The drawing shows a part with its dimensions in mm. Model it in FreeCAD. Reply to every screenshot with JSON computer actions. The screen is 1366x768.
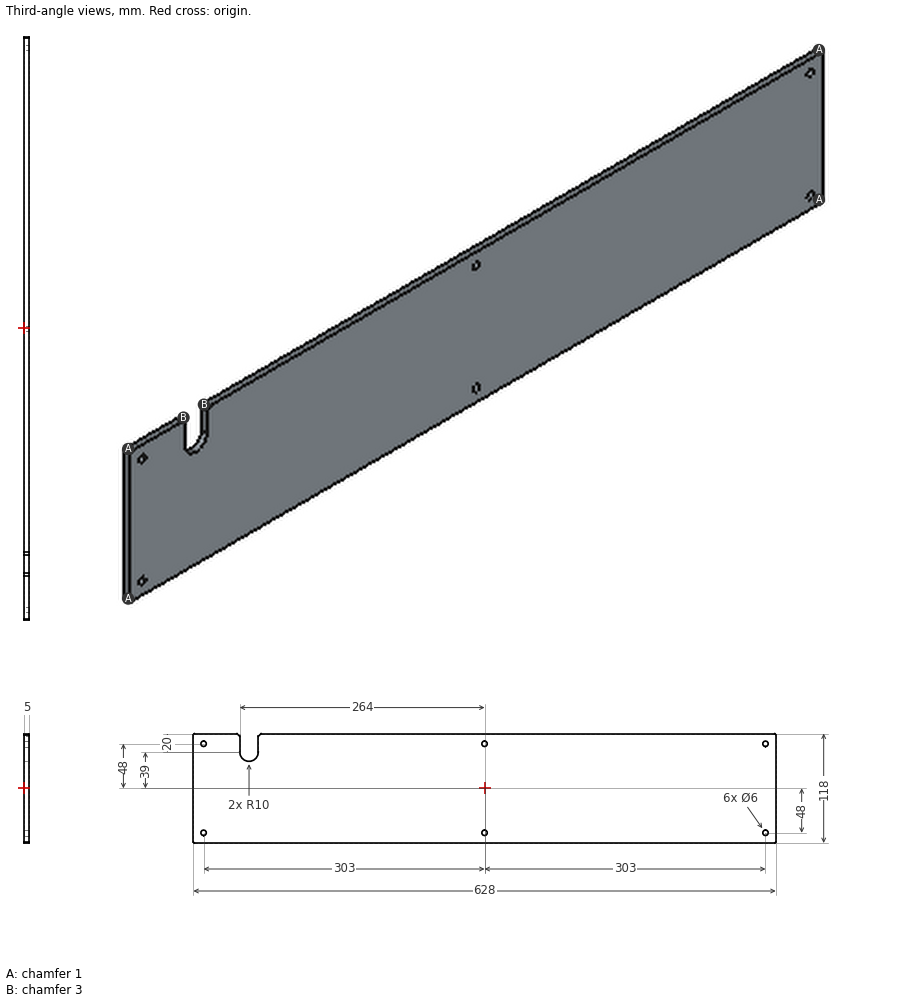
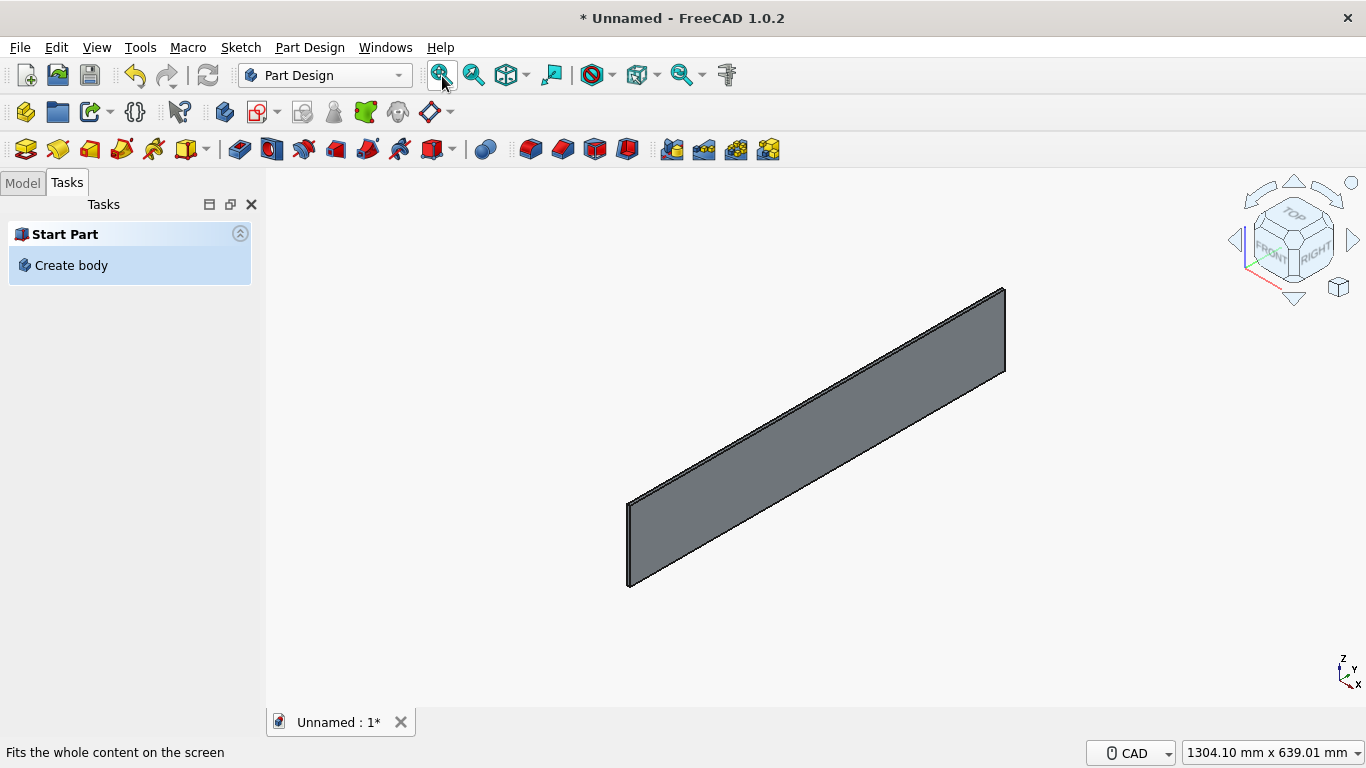
{"action": "key", "text": "2"}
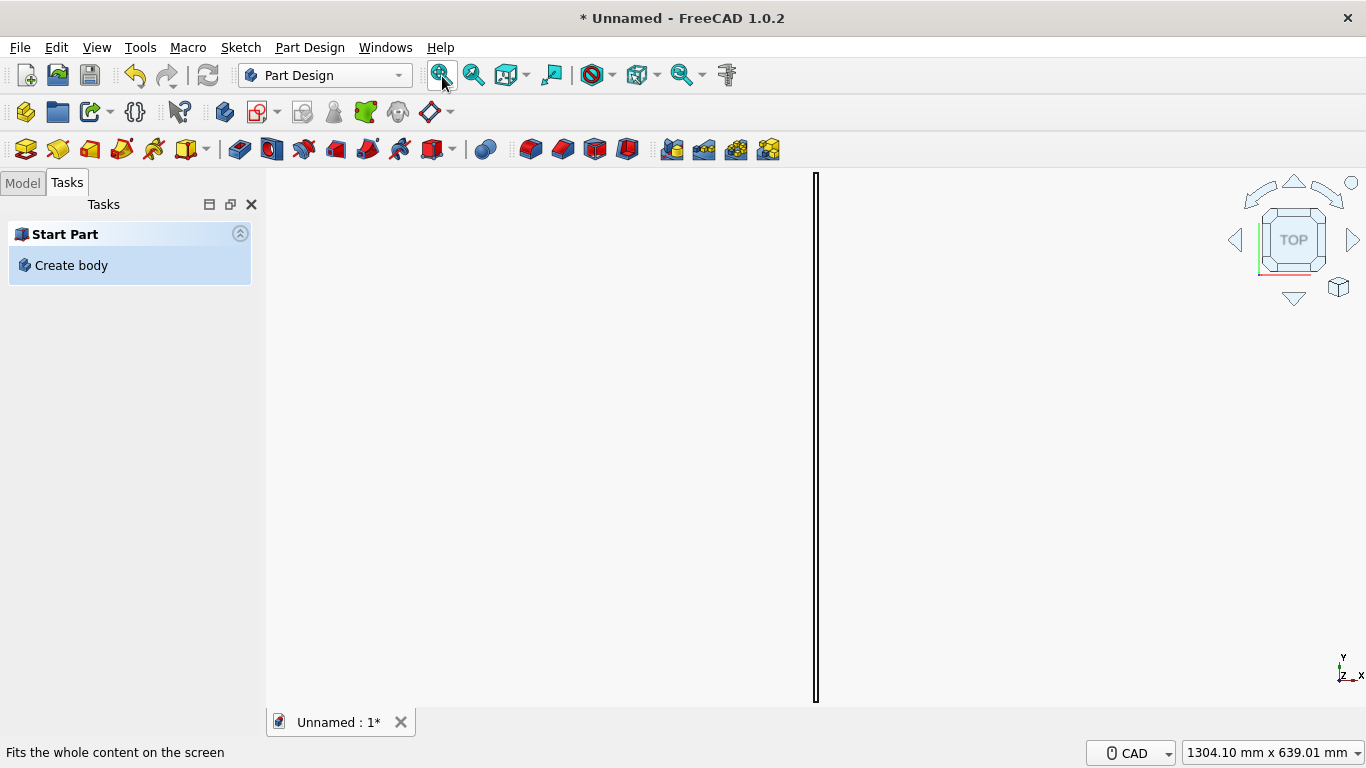
{"action": "key", "text": "1"}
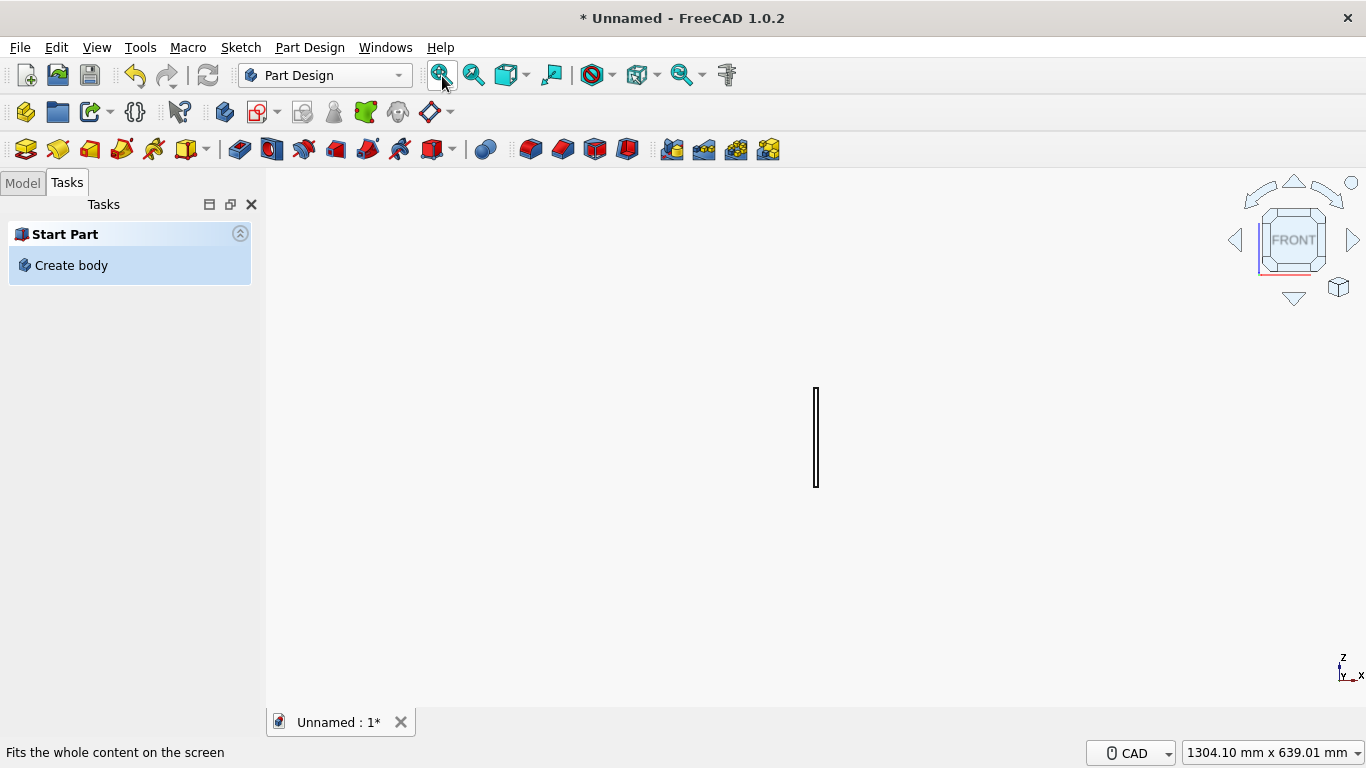
{"action": "key", "text": "v f"}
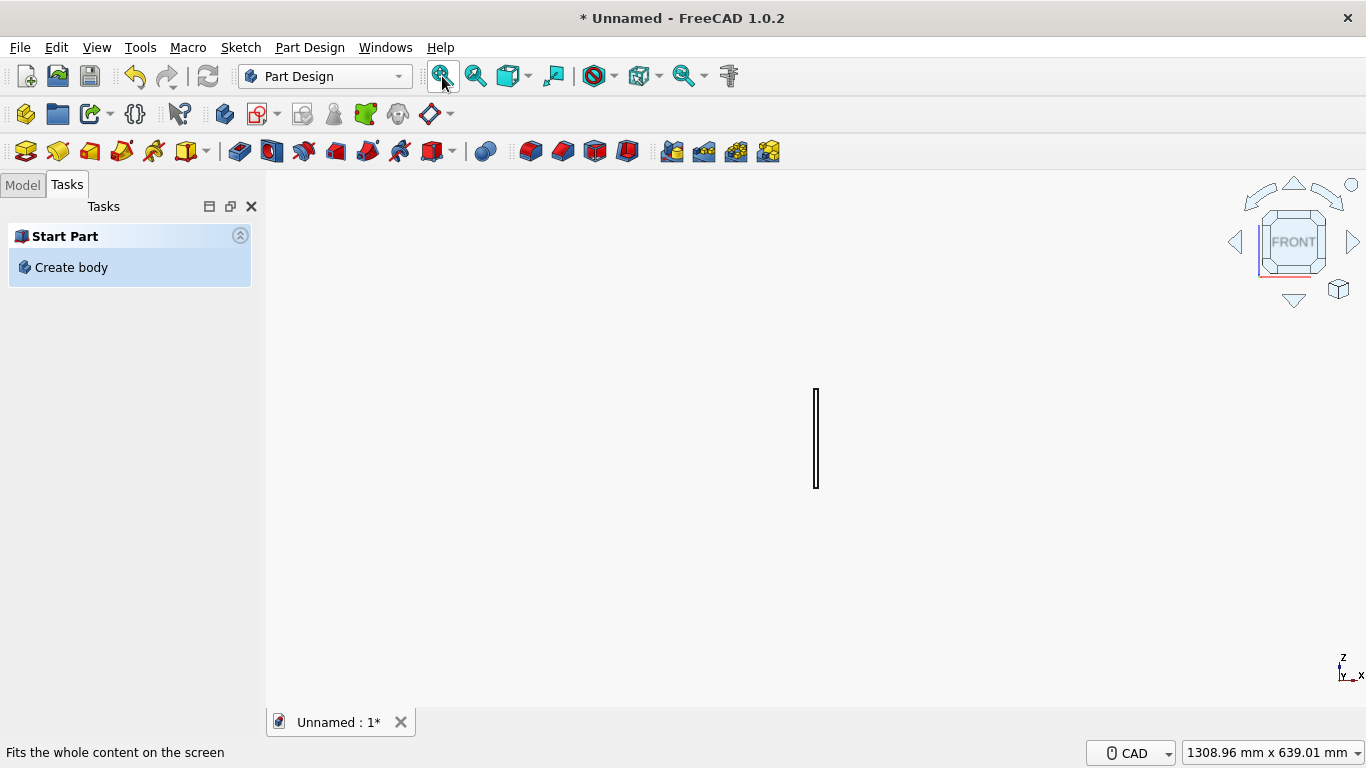
{"action": "scroll", "coordinate": [816, 388], "scroll_direction": "up", "scroll_amount": 12}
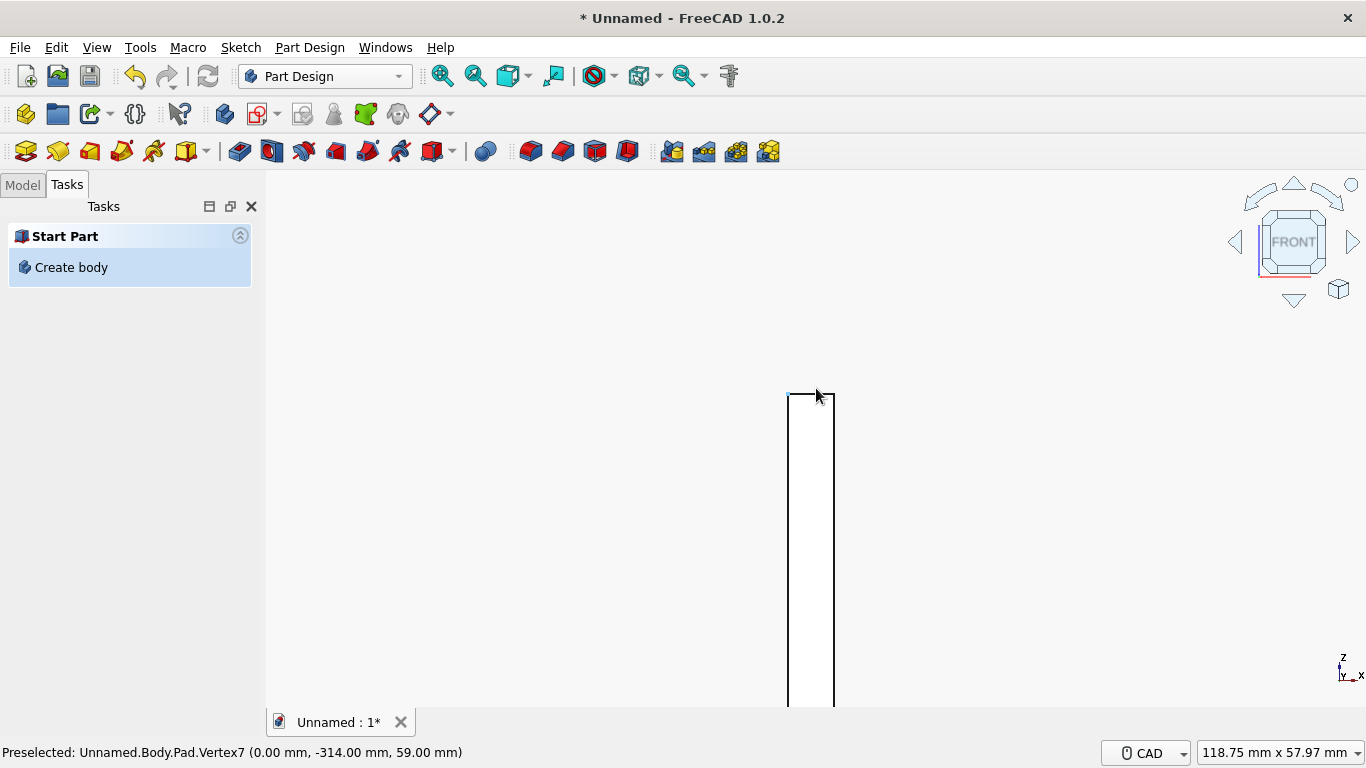
{"action": "left_click", "coordinate": [811, 393]}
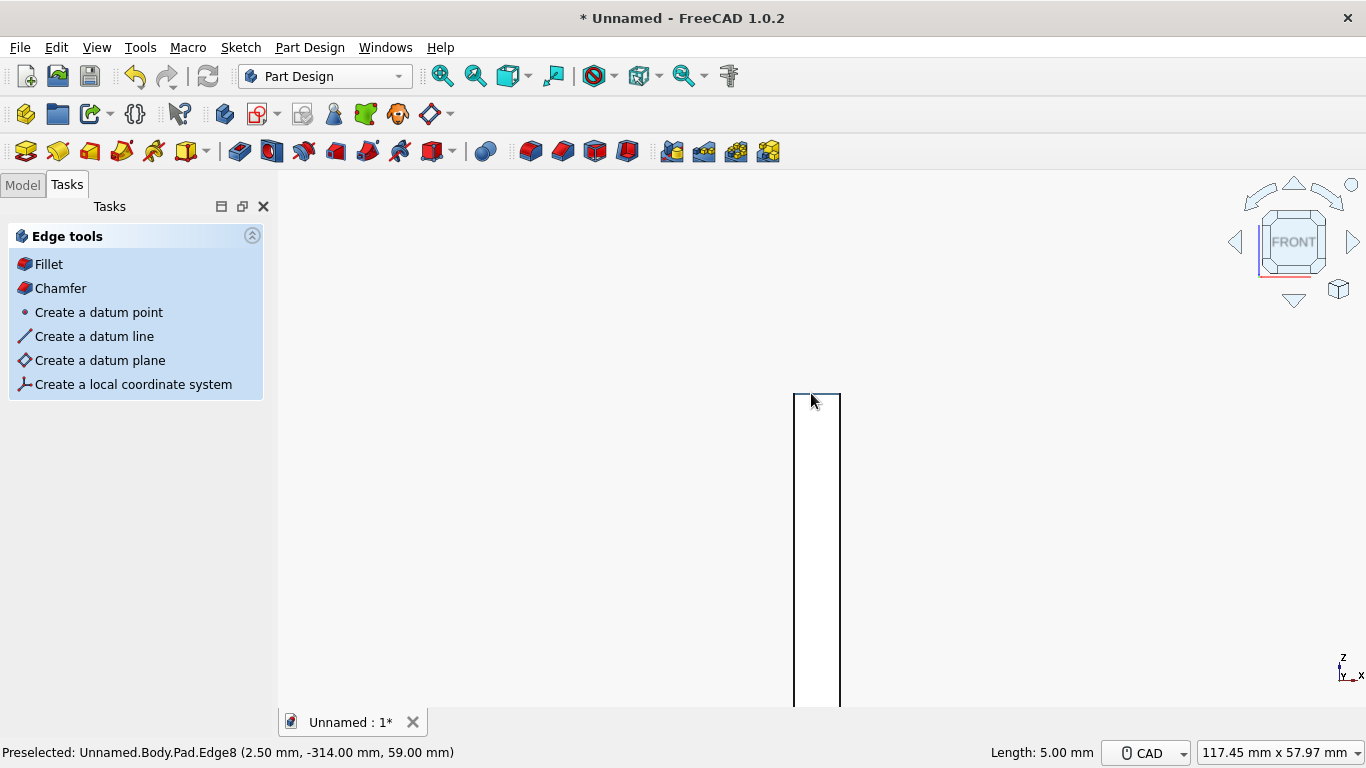
{"action": "left_click", "coordinate": [444, 76]}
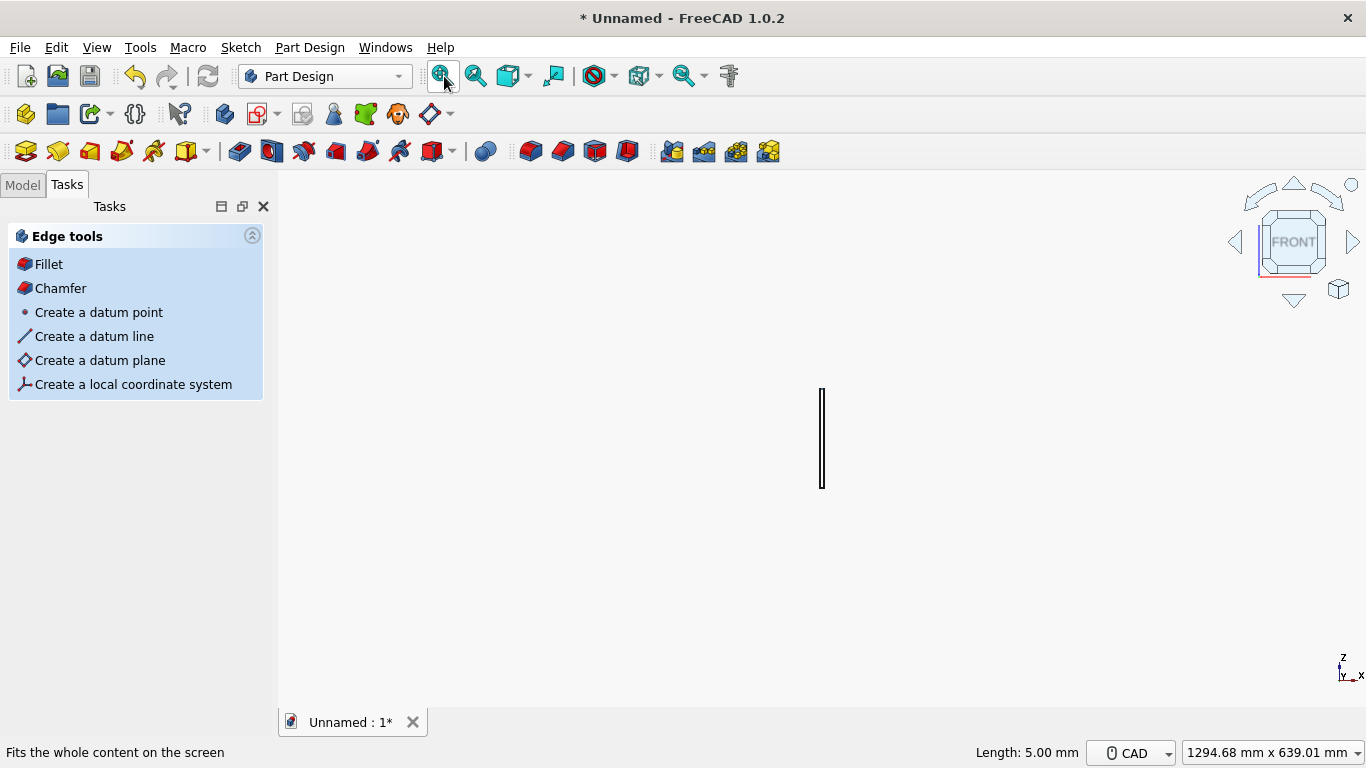
{"action": "key", "text": "3"}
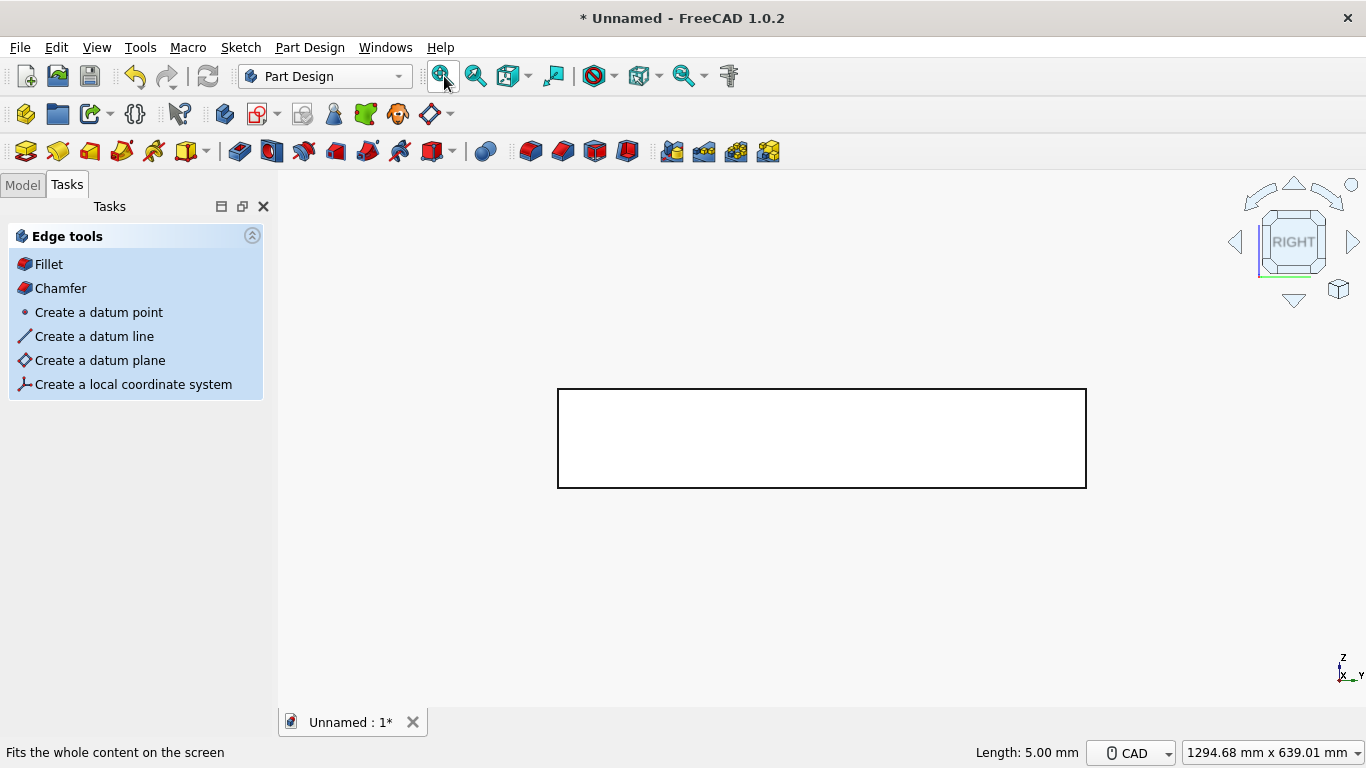
{"action": "scroll", "coordinate": [1086, 388], "scroll_direction": "up", "scroll_amount": 12}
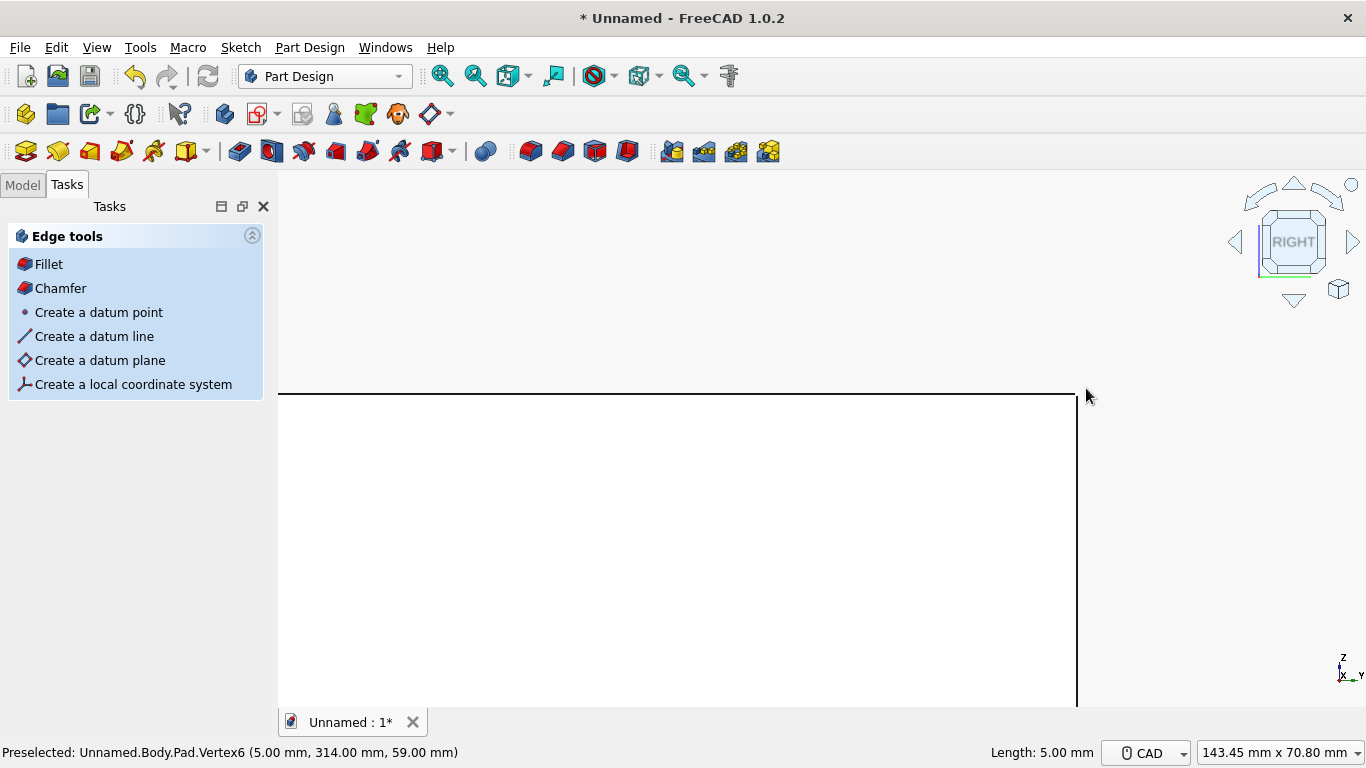
{"action": "left_click", "coordinate": [444, 76]}